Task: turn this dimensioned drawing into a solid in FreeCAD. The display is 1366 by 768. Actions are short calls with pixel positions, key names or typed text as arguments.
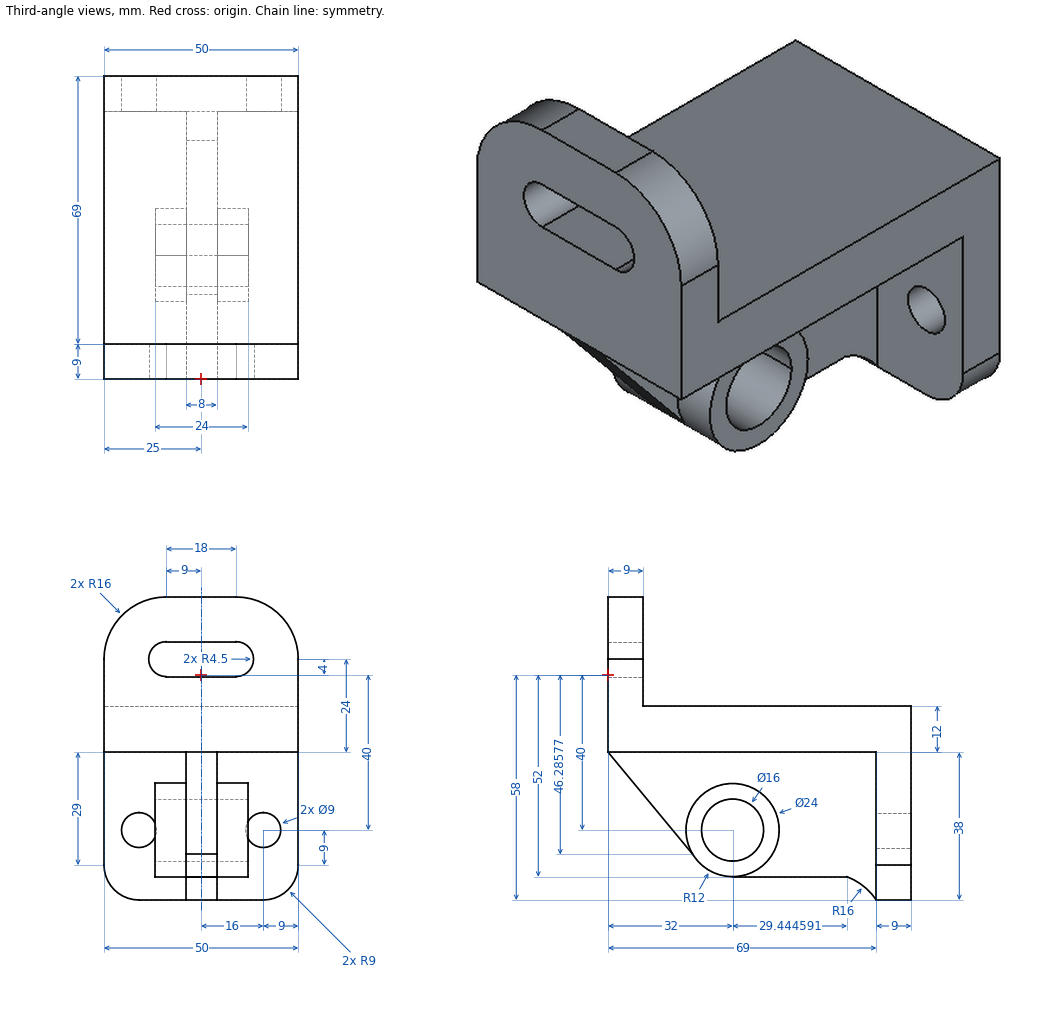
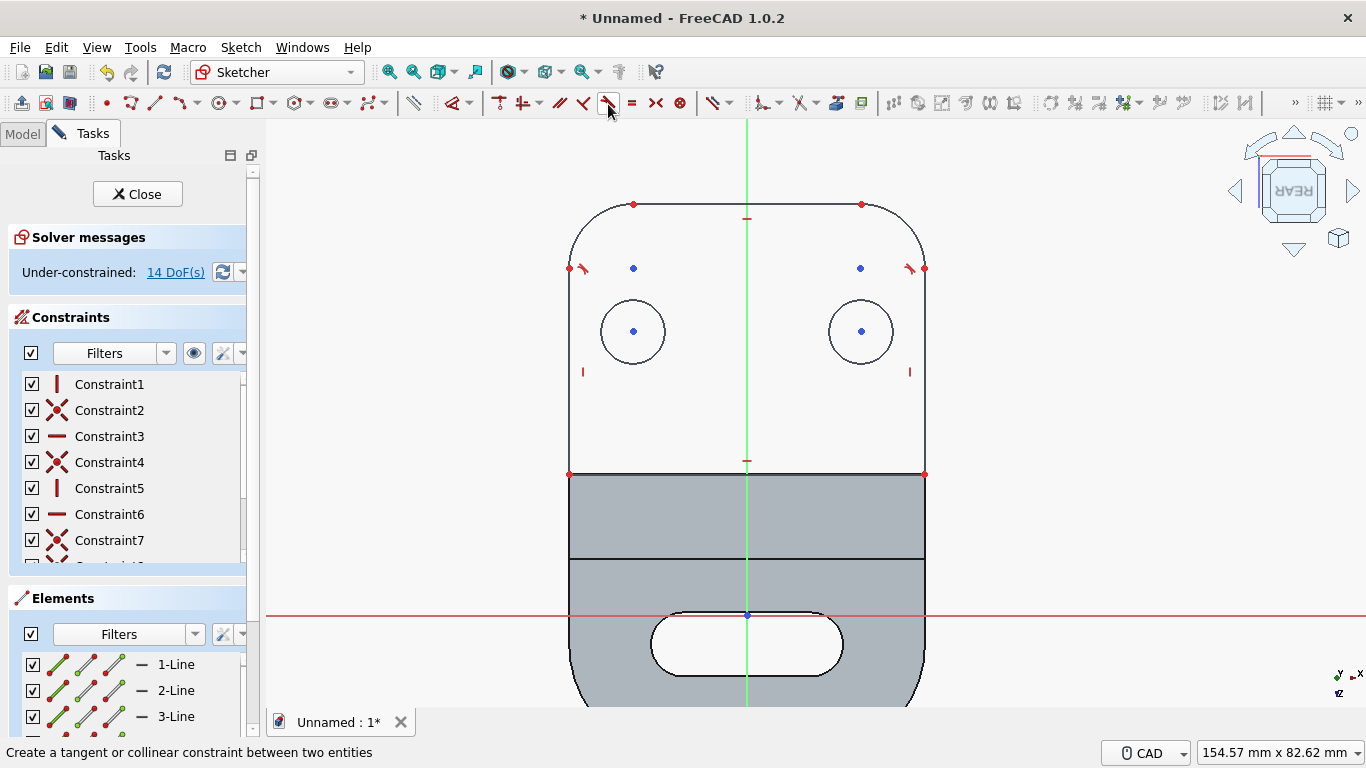
click(793, 204)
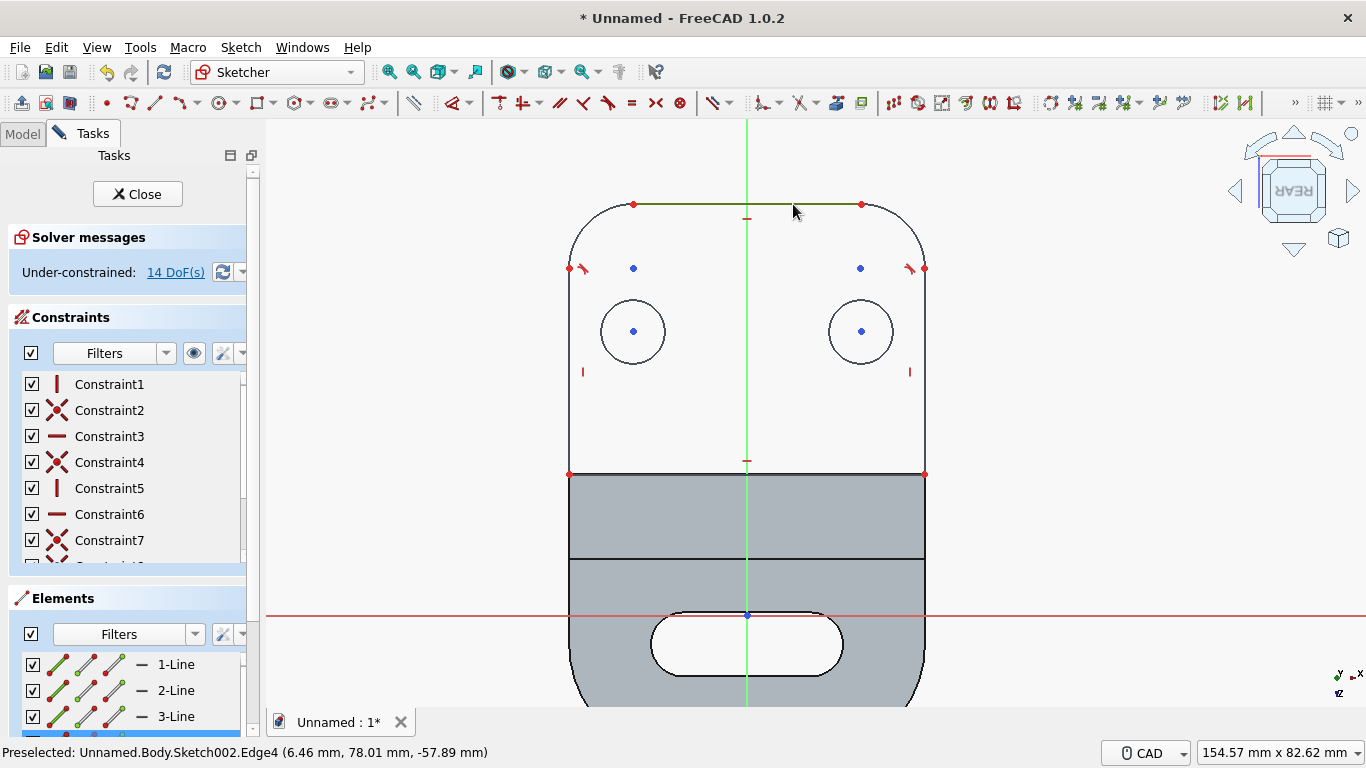
click(918, 240)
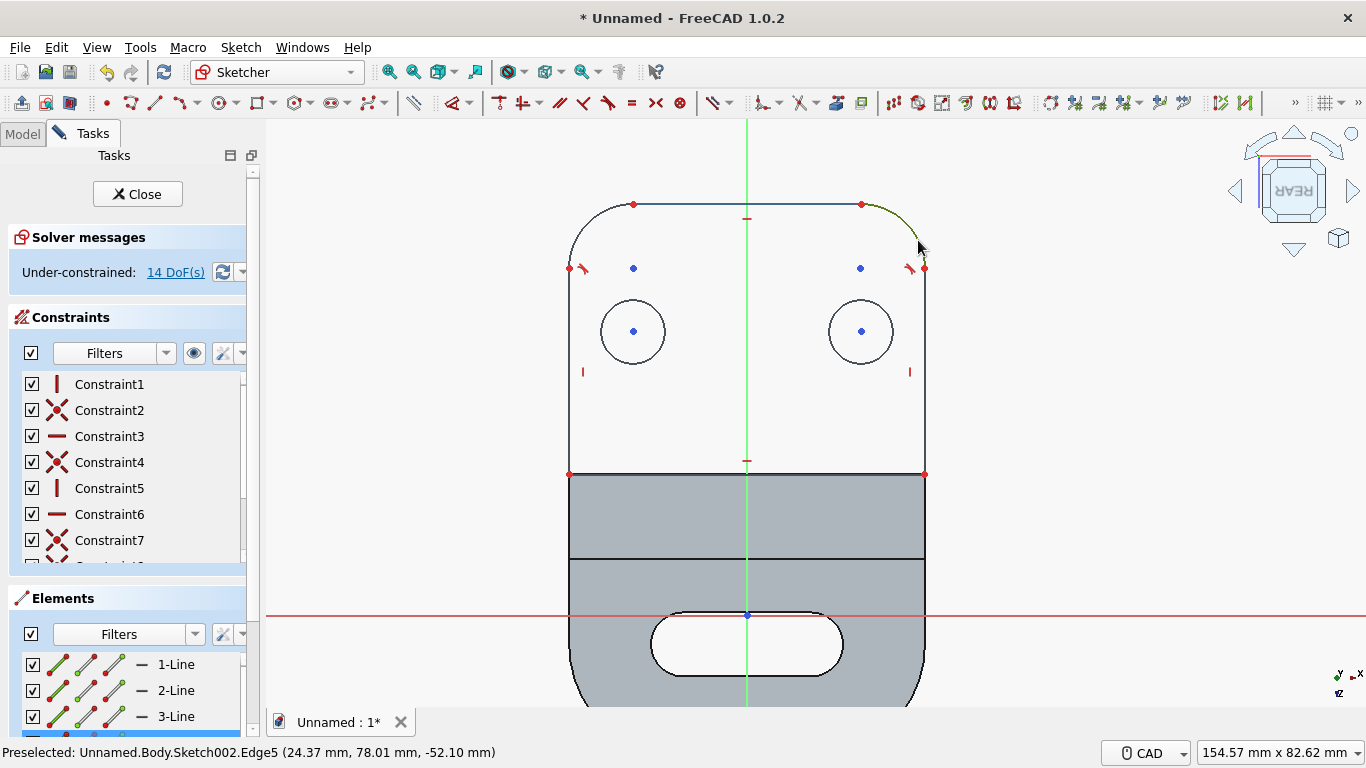
click(608, 104)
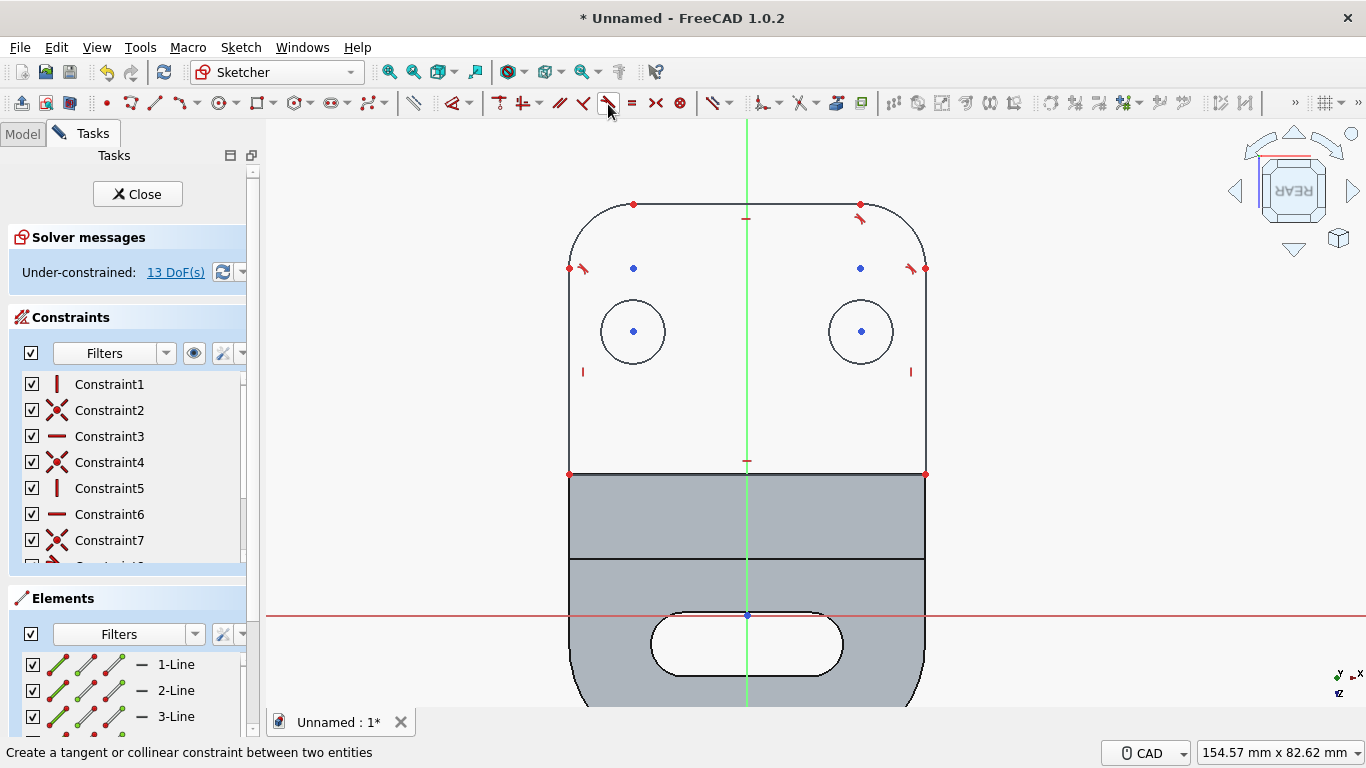
click(793, 204)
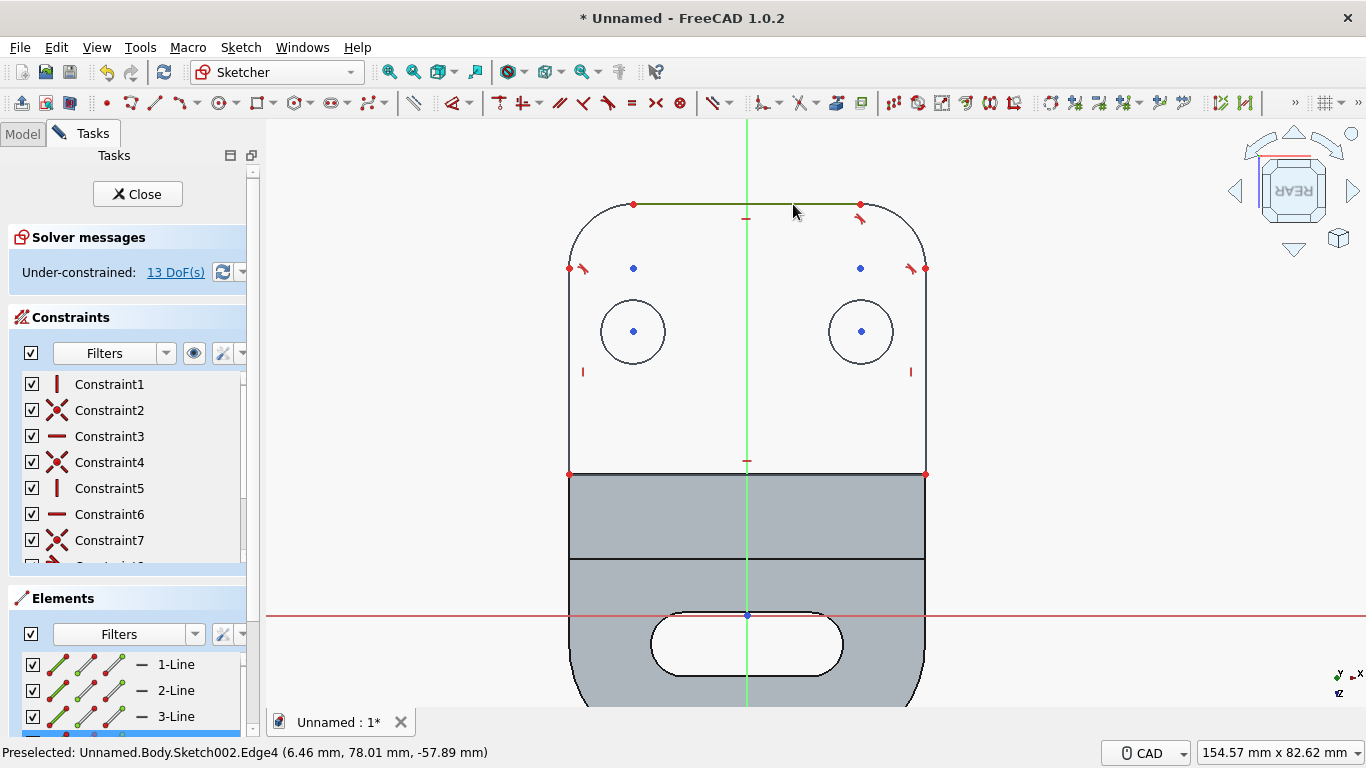
click(604, 211)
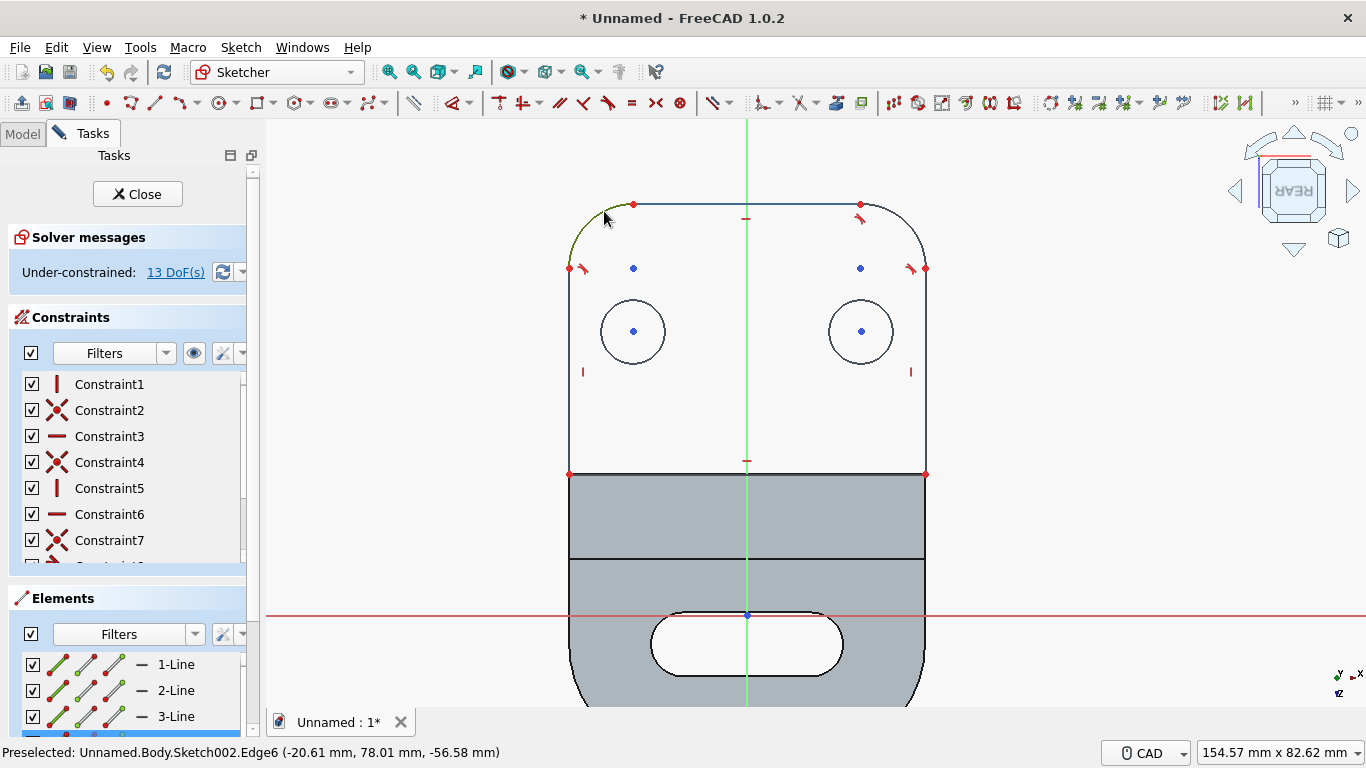
key(t)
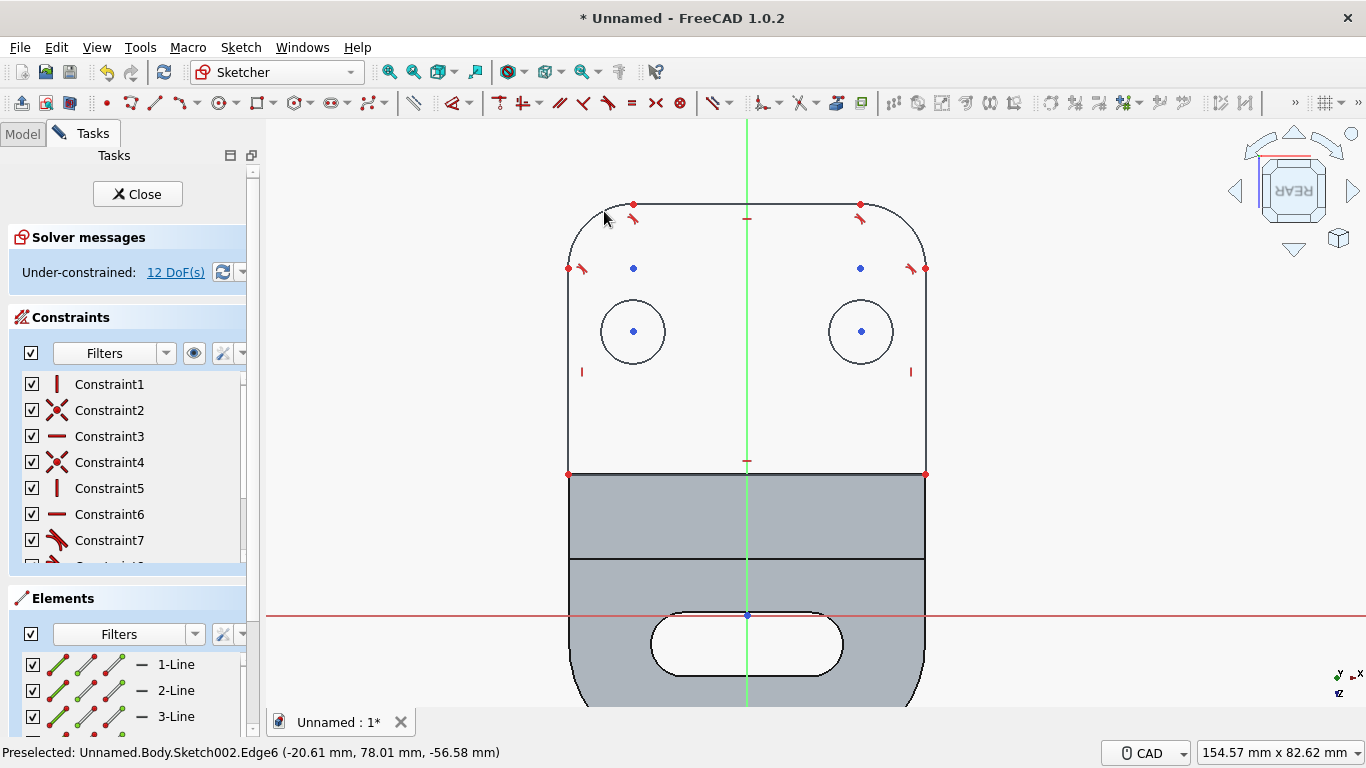
click(919, 239)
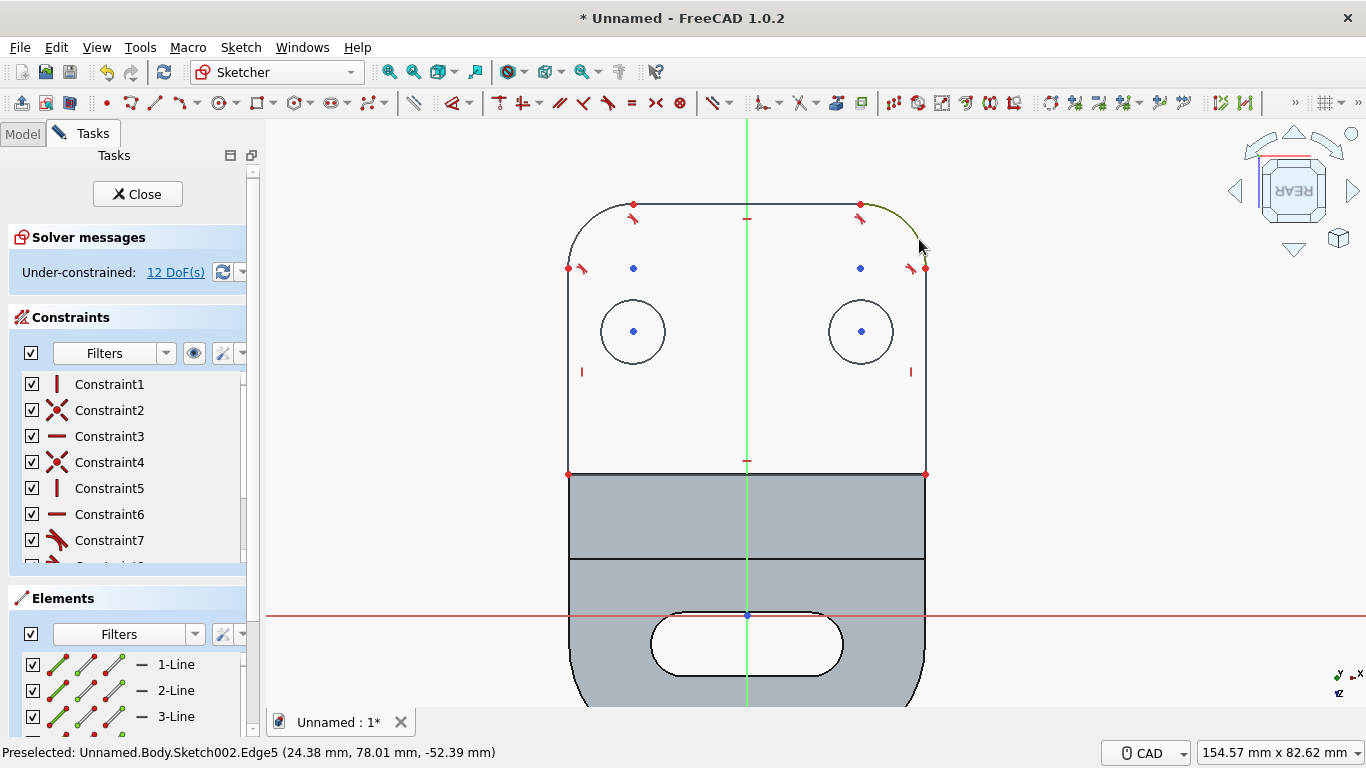
click(604, 211)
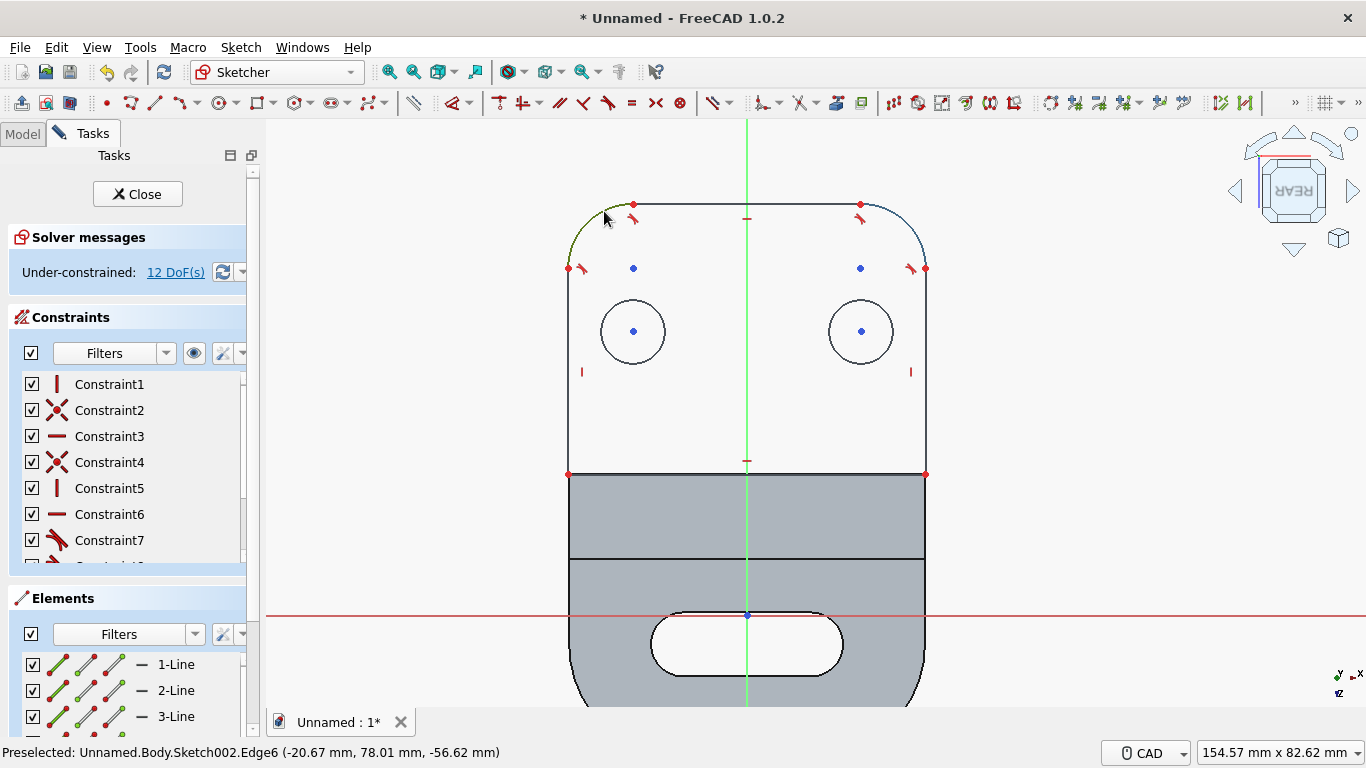
key(e)